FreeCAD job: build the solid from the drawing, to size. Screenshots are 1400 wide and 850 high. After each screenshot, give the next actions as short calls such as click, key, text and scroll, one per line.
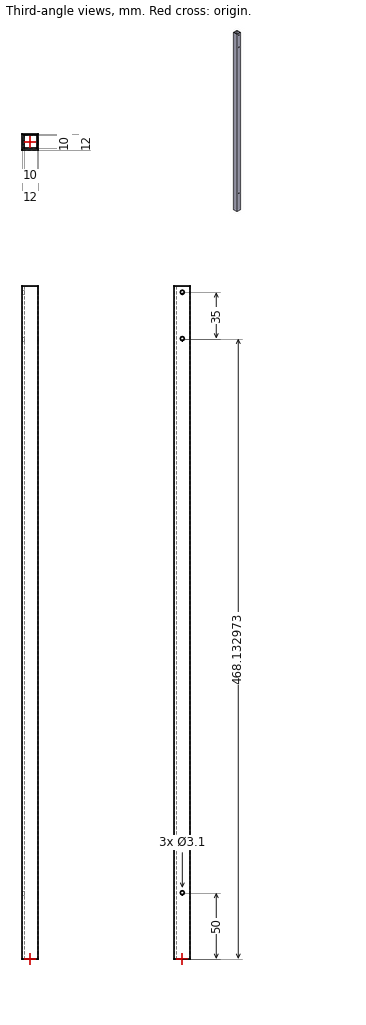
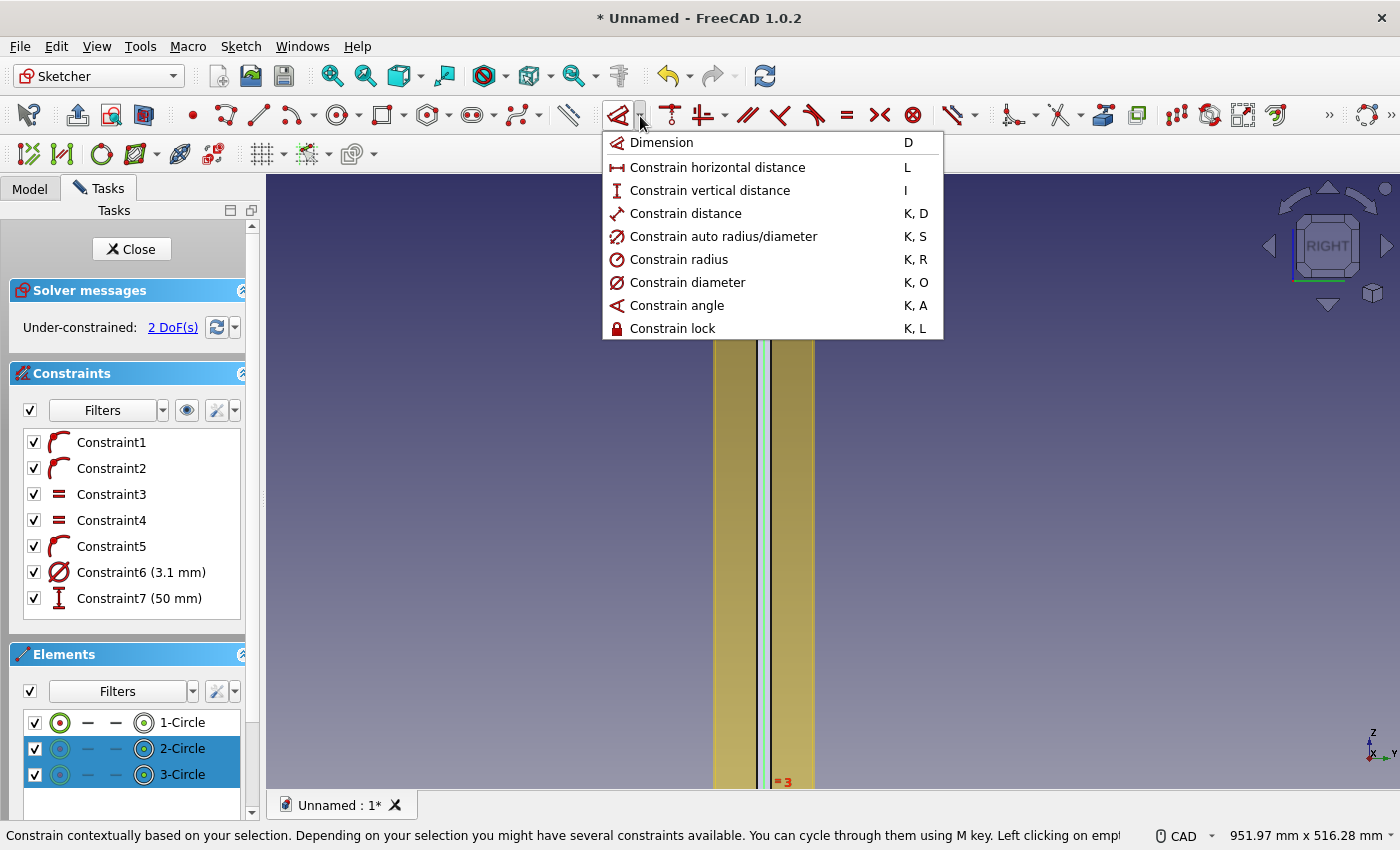
click(773, 190)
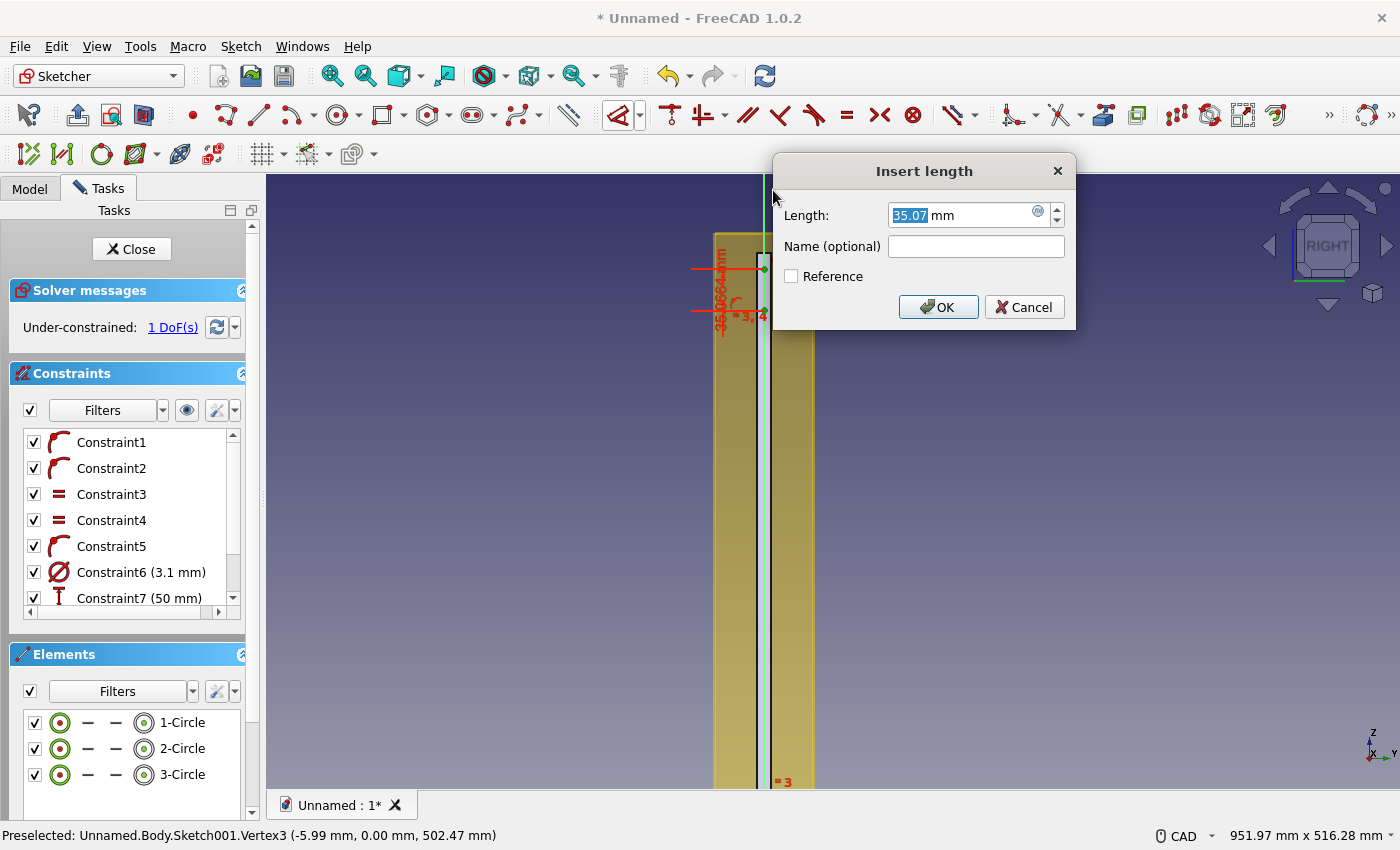
text(35)
key(Return)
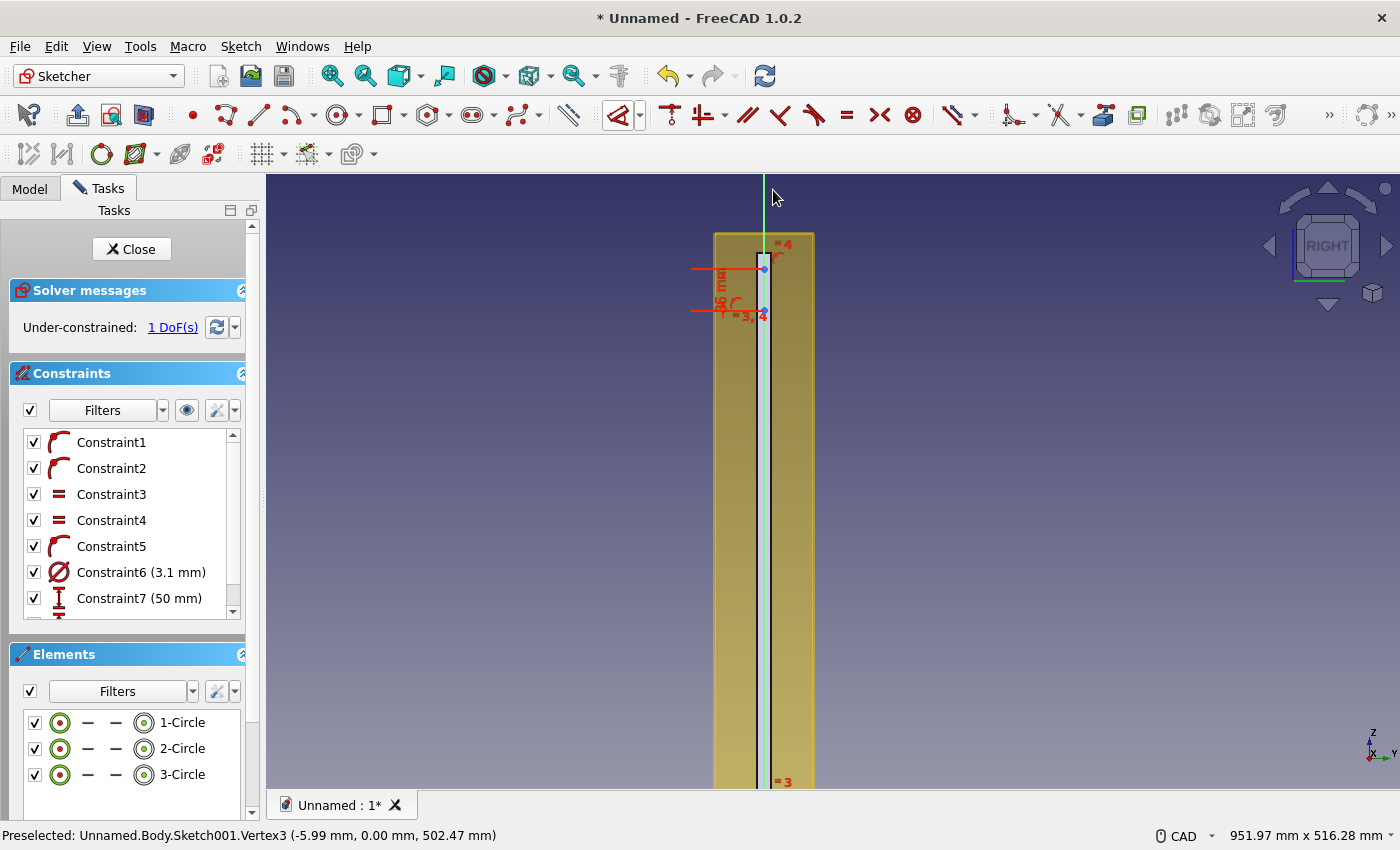
click(764, 311)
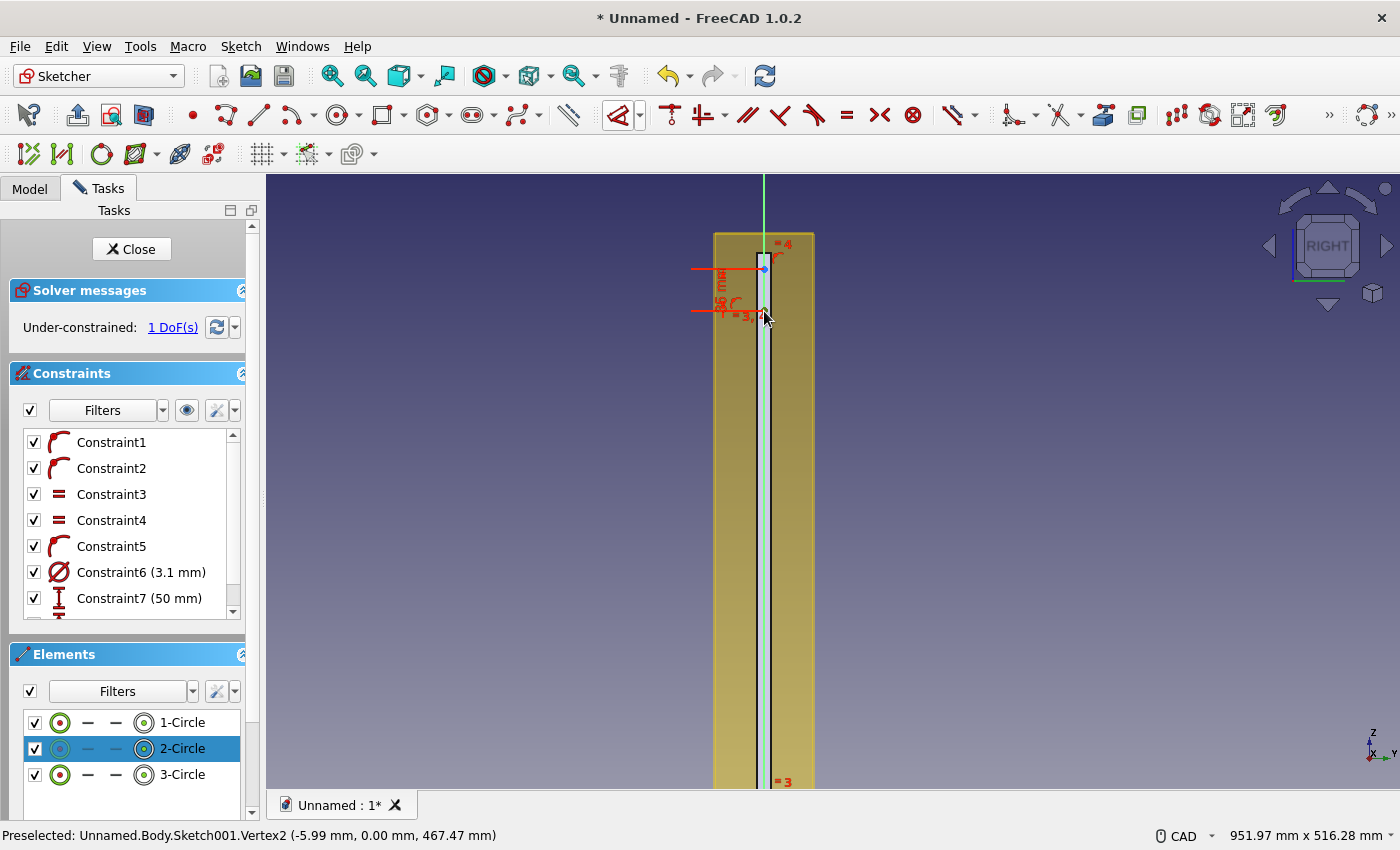
click(640, 116)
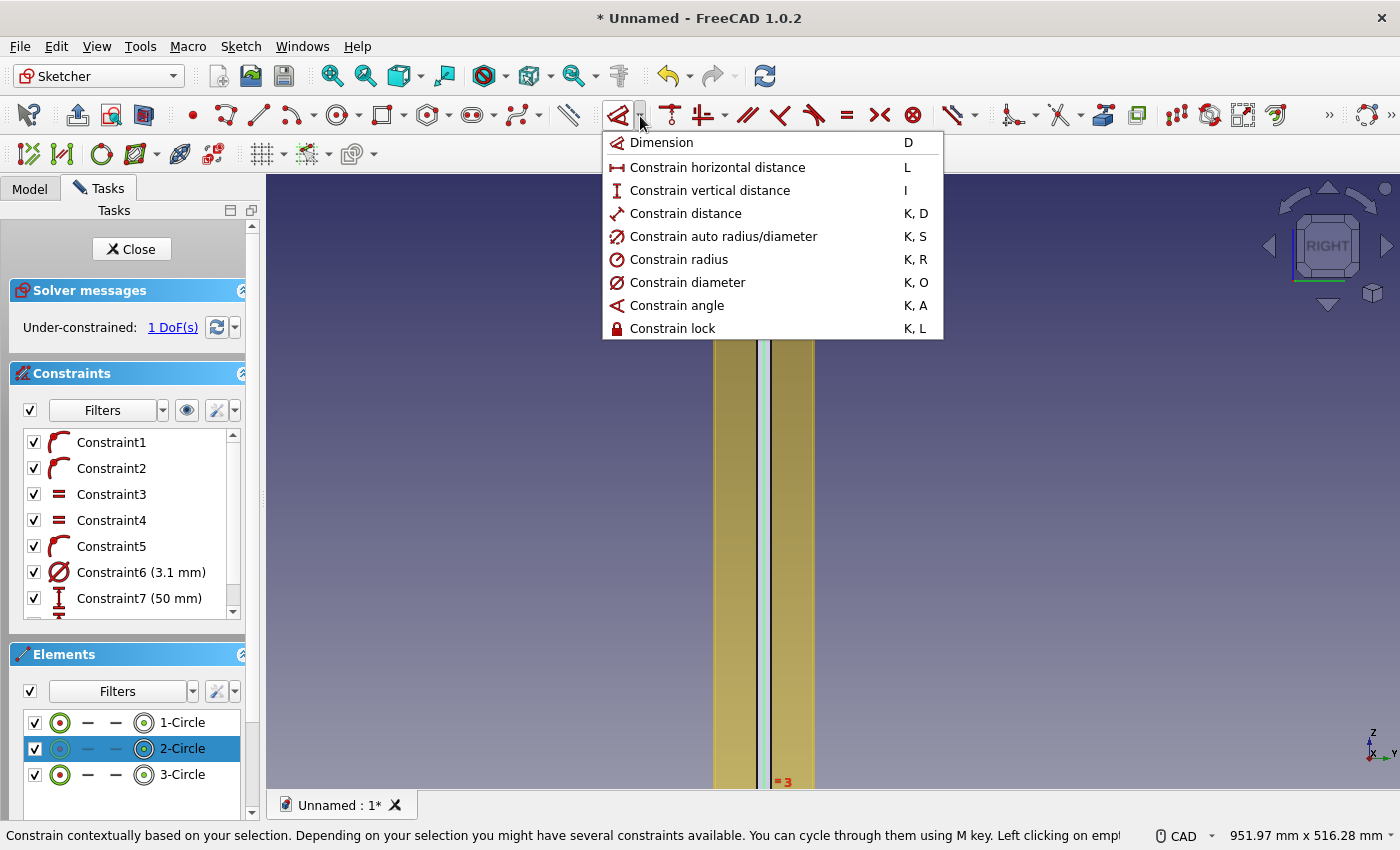
click(773, 190)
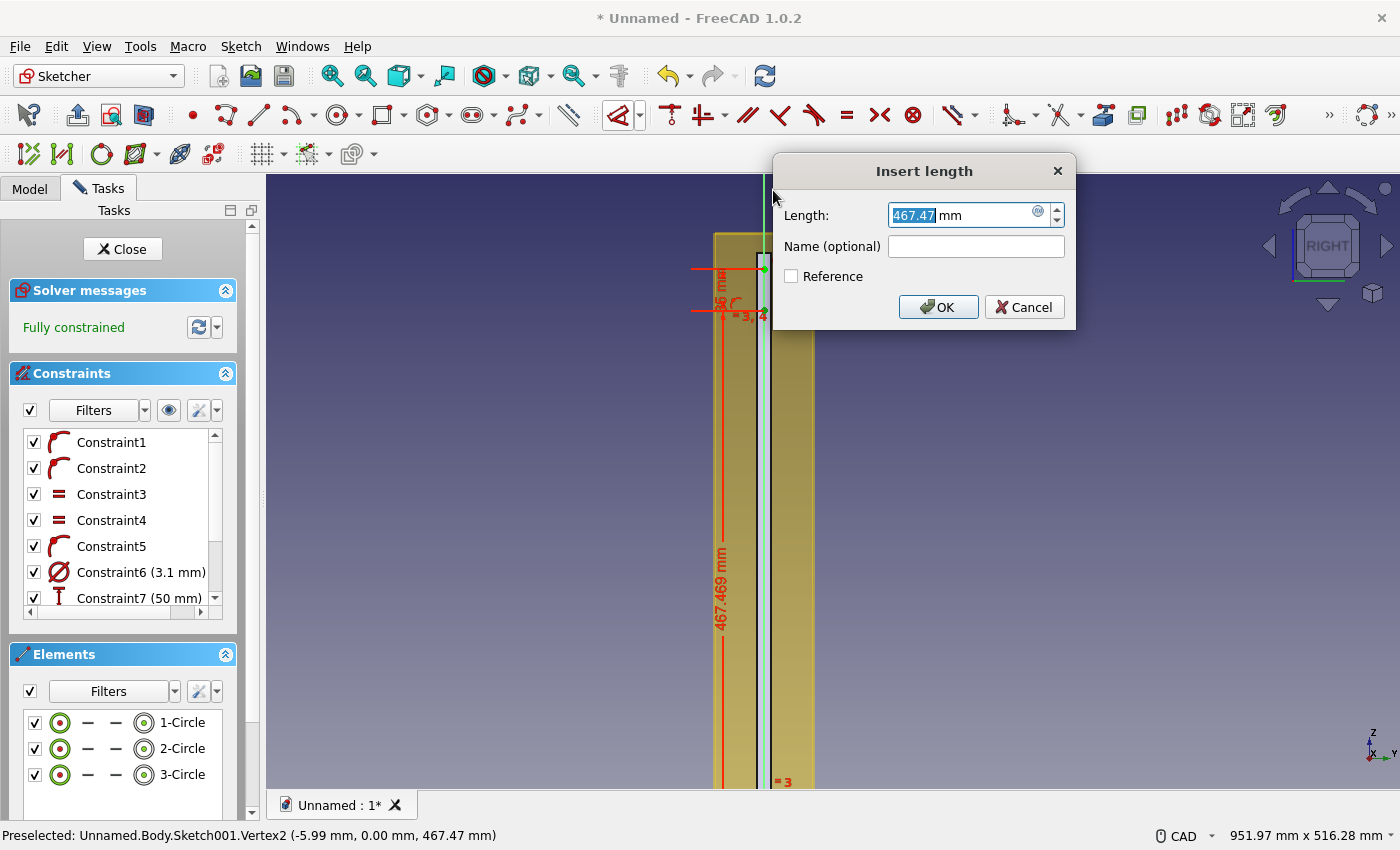
text(468.132973)
key(Return)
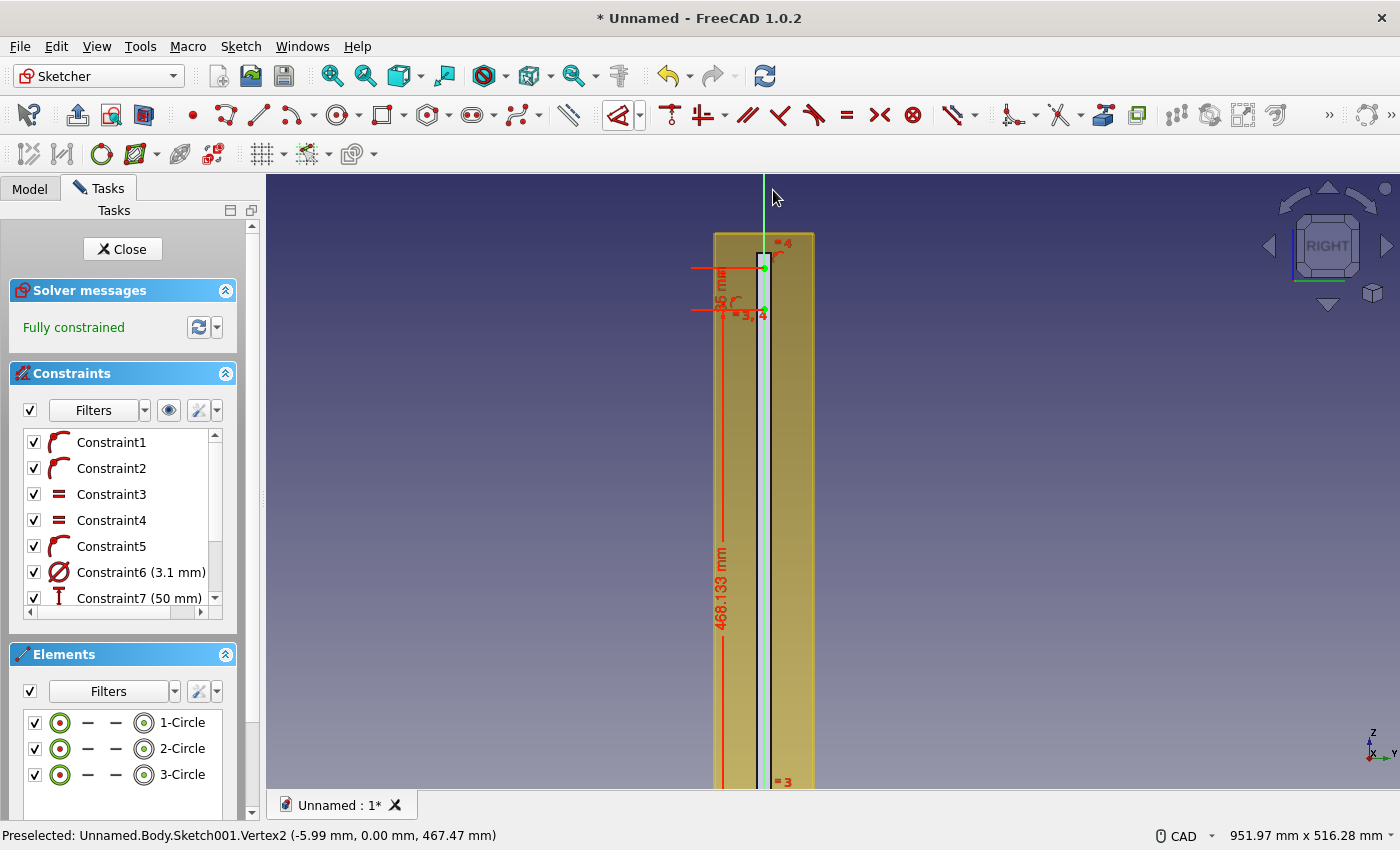
click(123, 249)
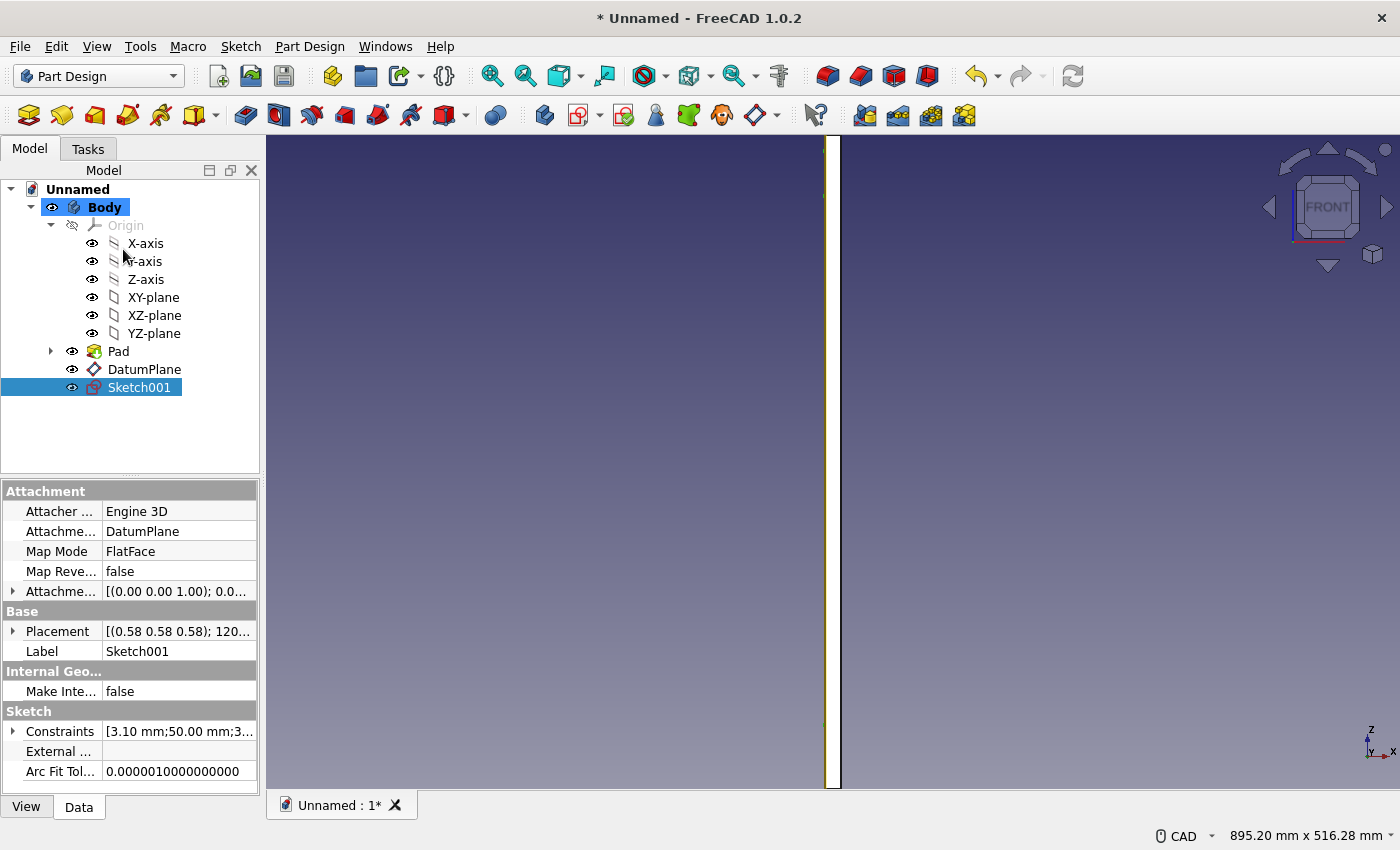
click(246, 116)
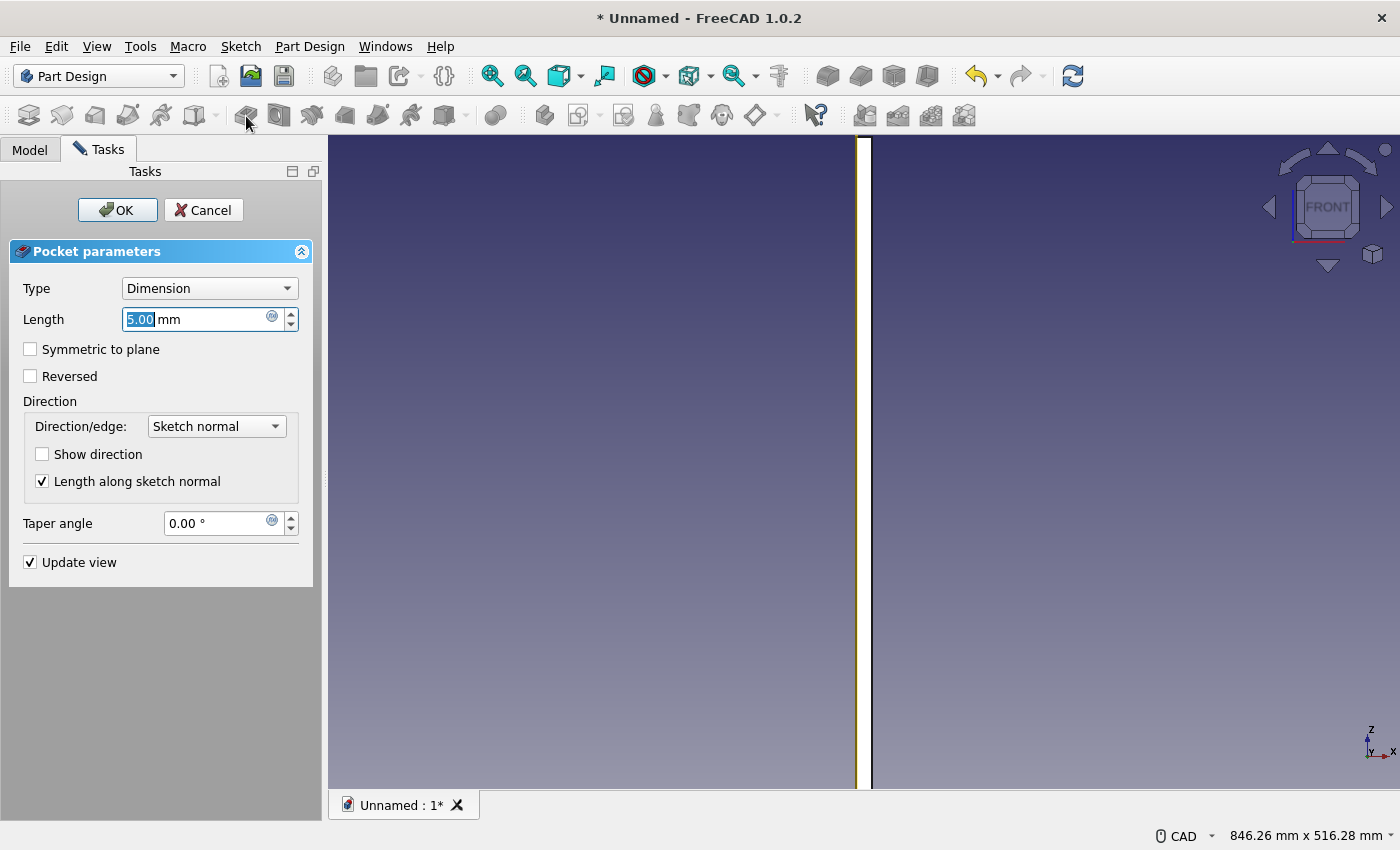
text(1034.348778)
key(Tab)